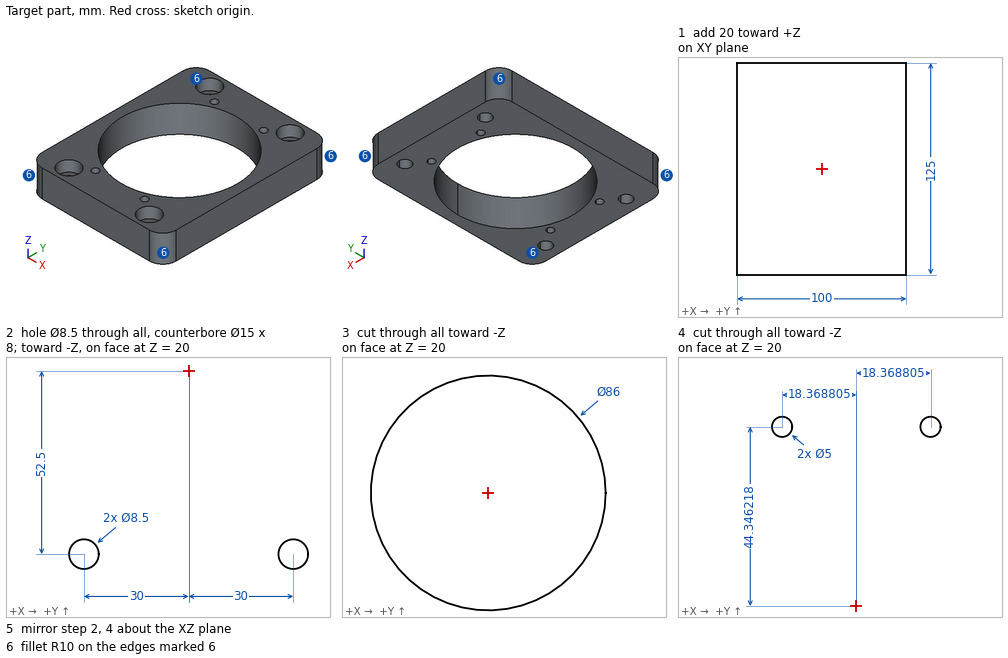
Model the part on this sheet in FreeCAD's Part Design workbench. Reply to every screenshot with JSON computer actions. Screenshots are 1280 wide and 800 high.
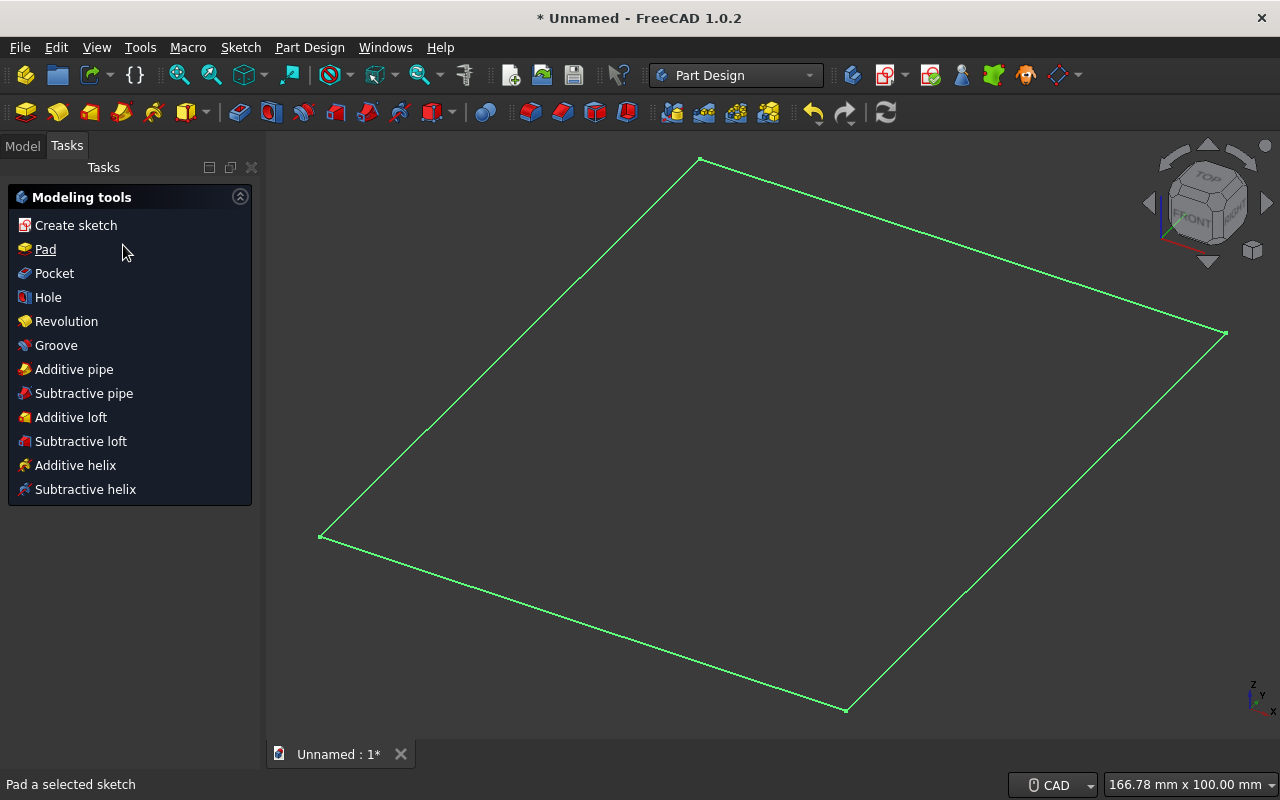
{"action": "left_click", "coordinate": [26, 112]}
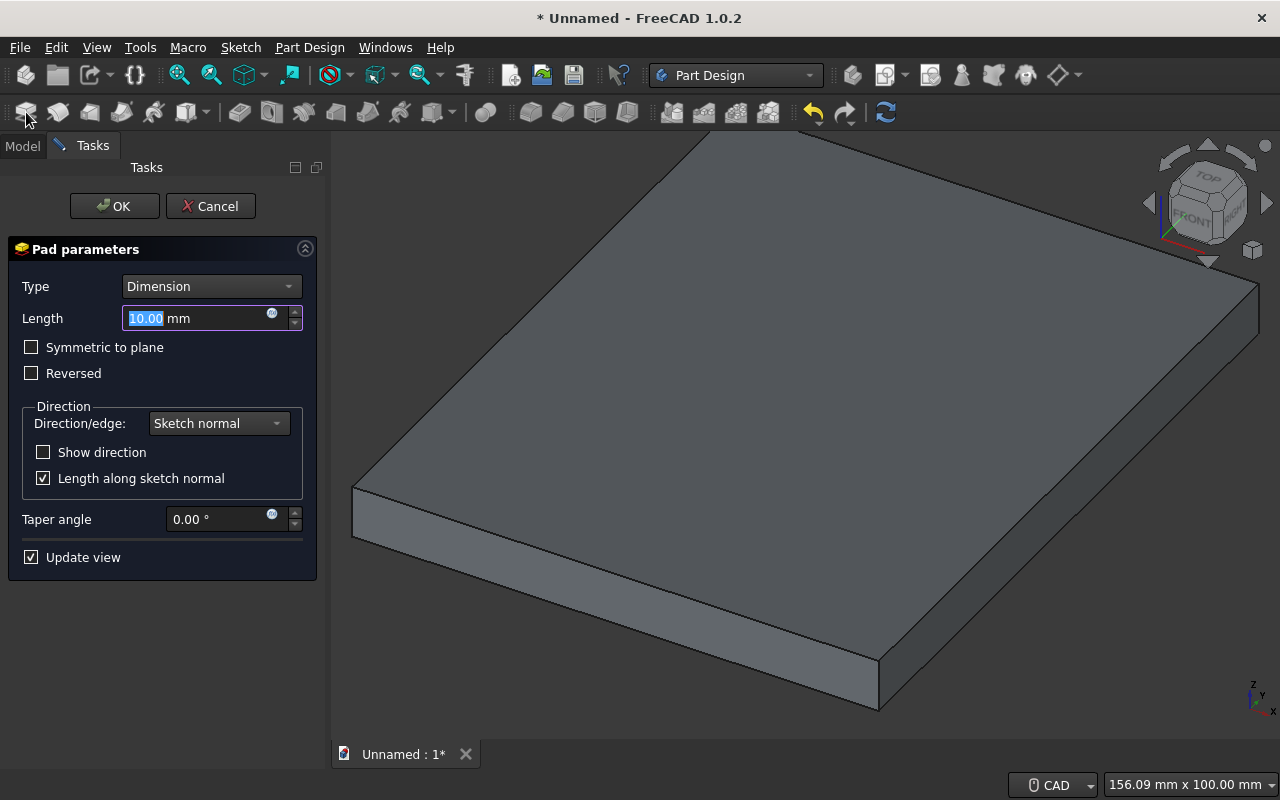
{"action": "type", "text": "20"}
{"action": "key", "text": "Tab"}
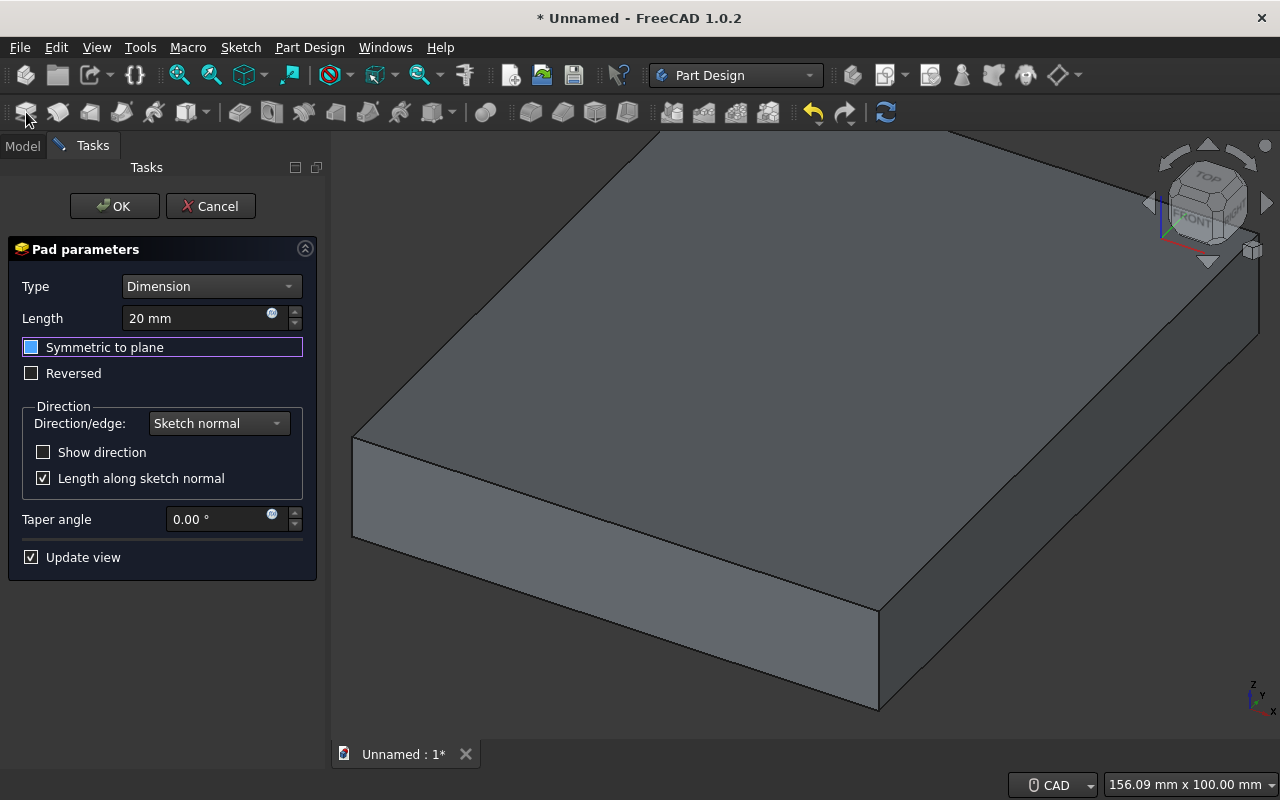
{"action": "left_click", "coordinate": [115, 206]}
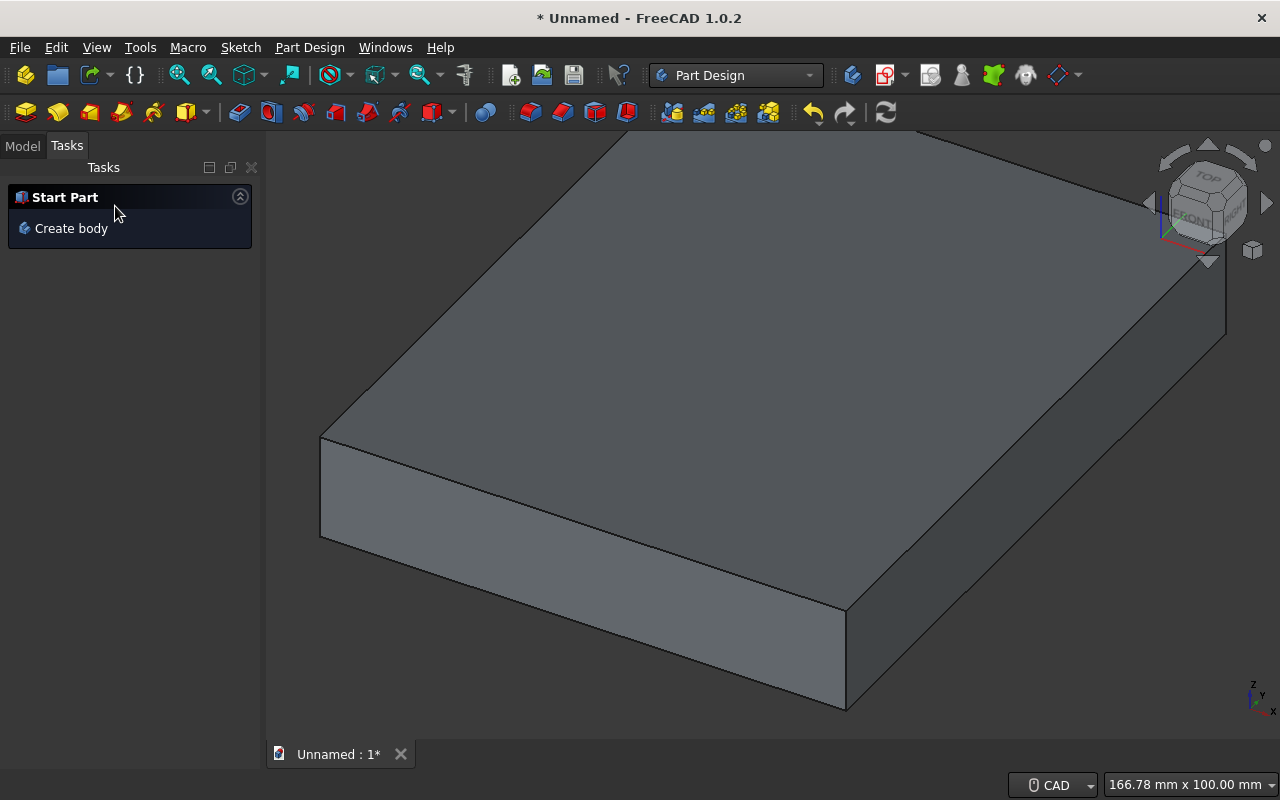
{"action": "left_click", "coordinate": [180, 76]}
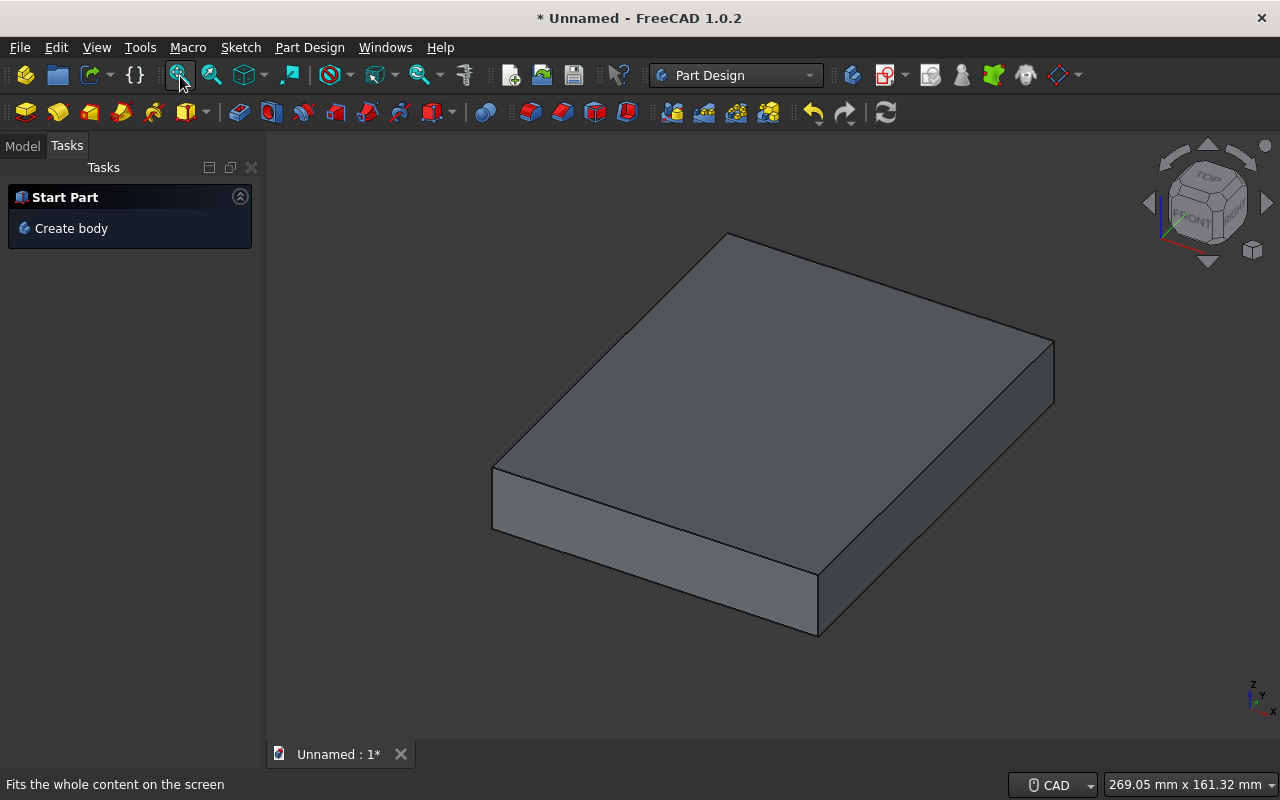
{"action": "left_click", "coordinate": [773, 403]}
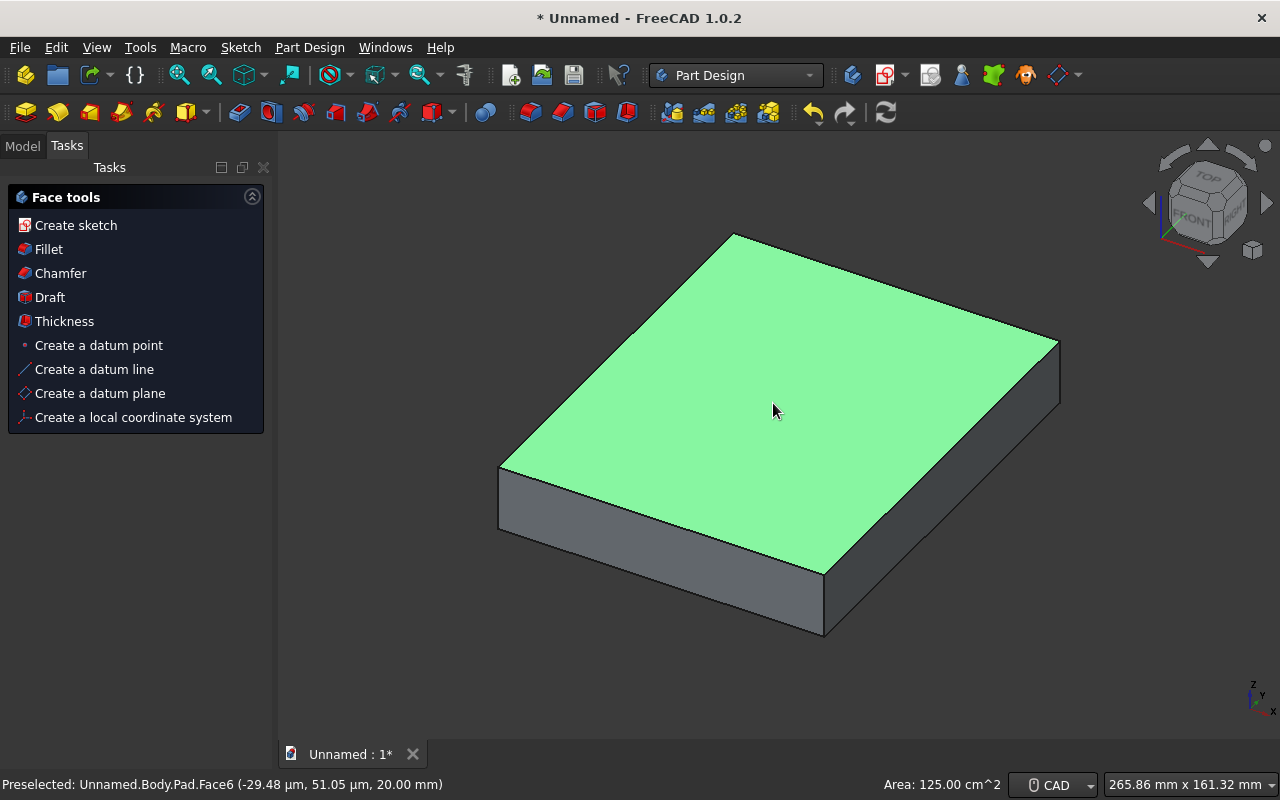
{"action": "left_click", "coordinate": [886, 76]}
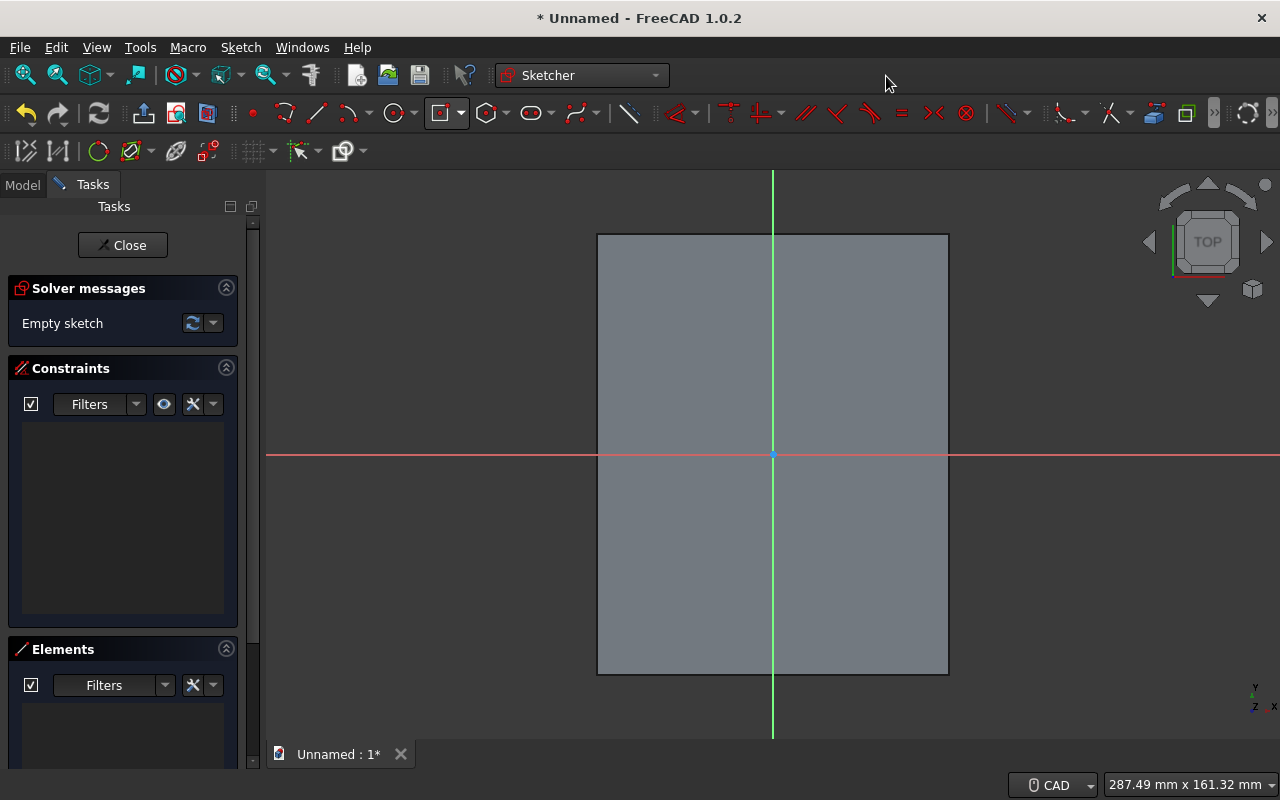
{"action": "scroll", "coordinate": [856, 676], "scroll_direction": "up", "scroll_amount": 3}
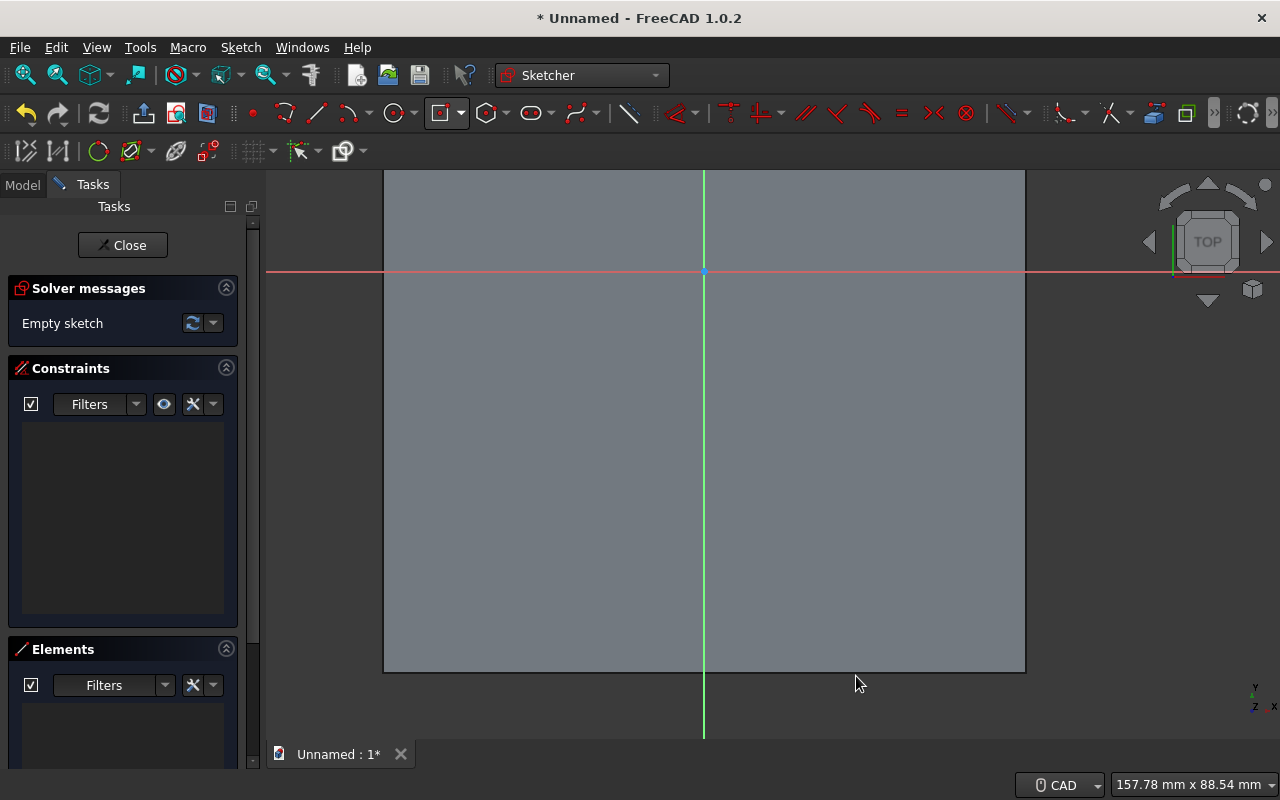
{"action": "left_click", "coordinate": [394, 114]}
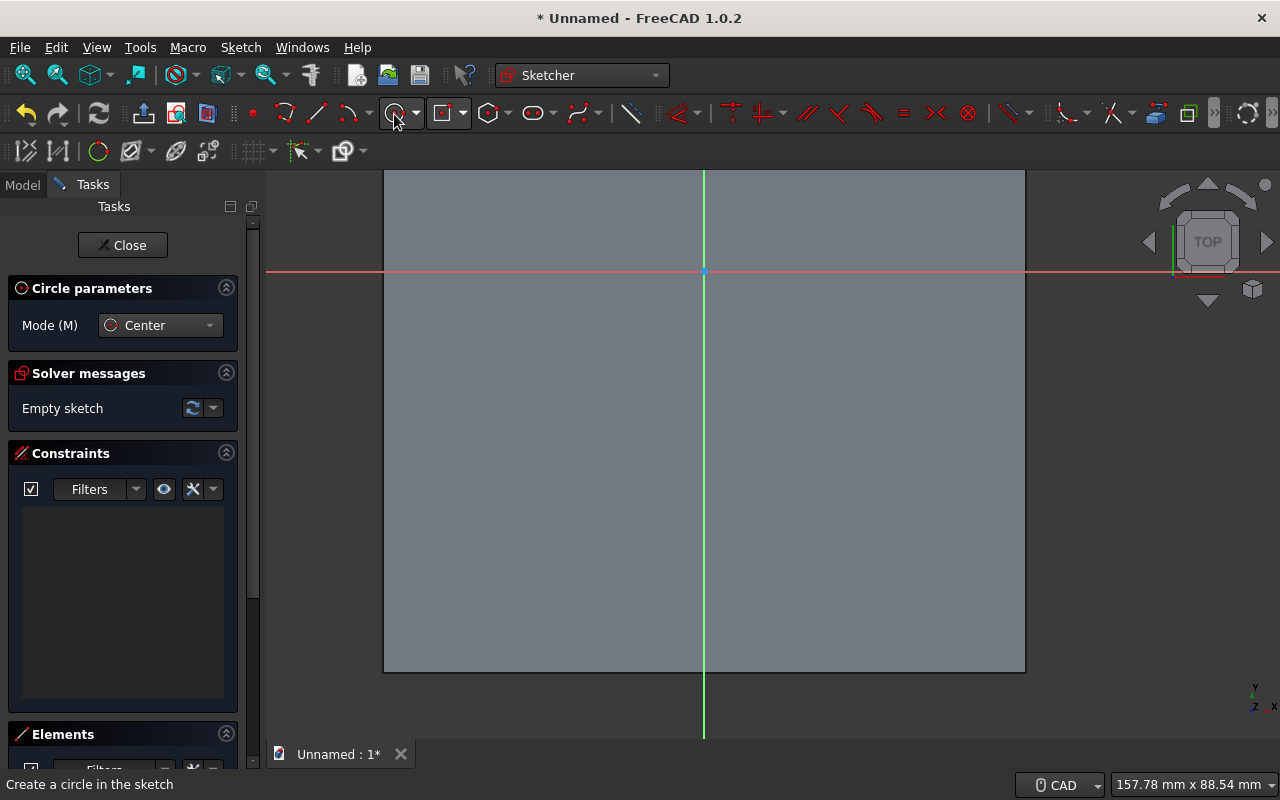
{"action": "left_click", "coordinate": [511, 609]}
{"action": "mouse_move", "coordinate": [531, 590]}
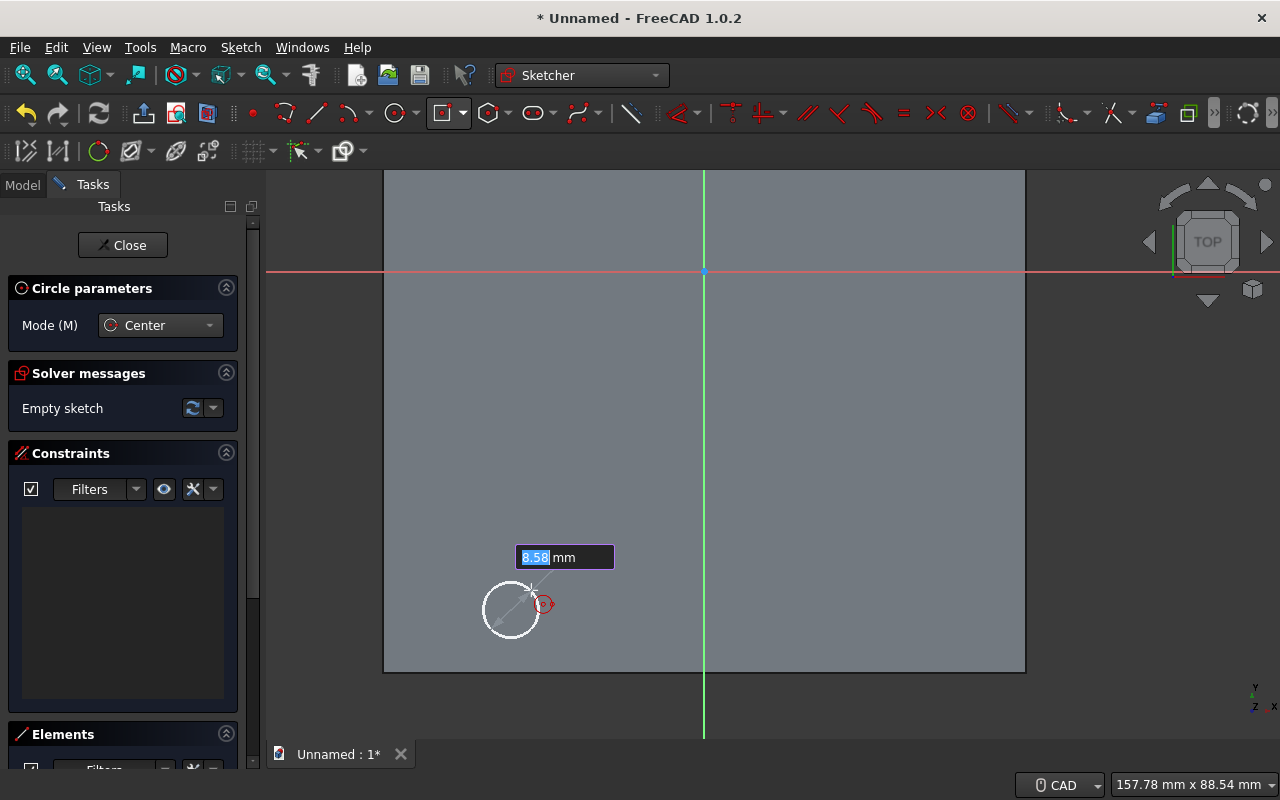
{"action": "type", "text": "8.5"}
{"action": "key", "text": "Return"}